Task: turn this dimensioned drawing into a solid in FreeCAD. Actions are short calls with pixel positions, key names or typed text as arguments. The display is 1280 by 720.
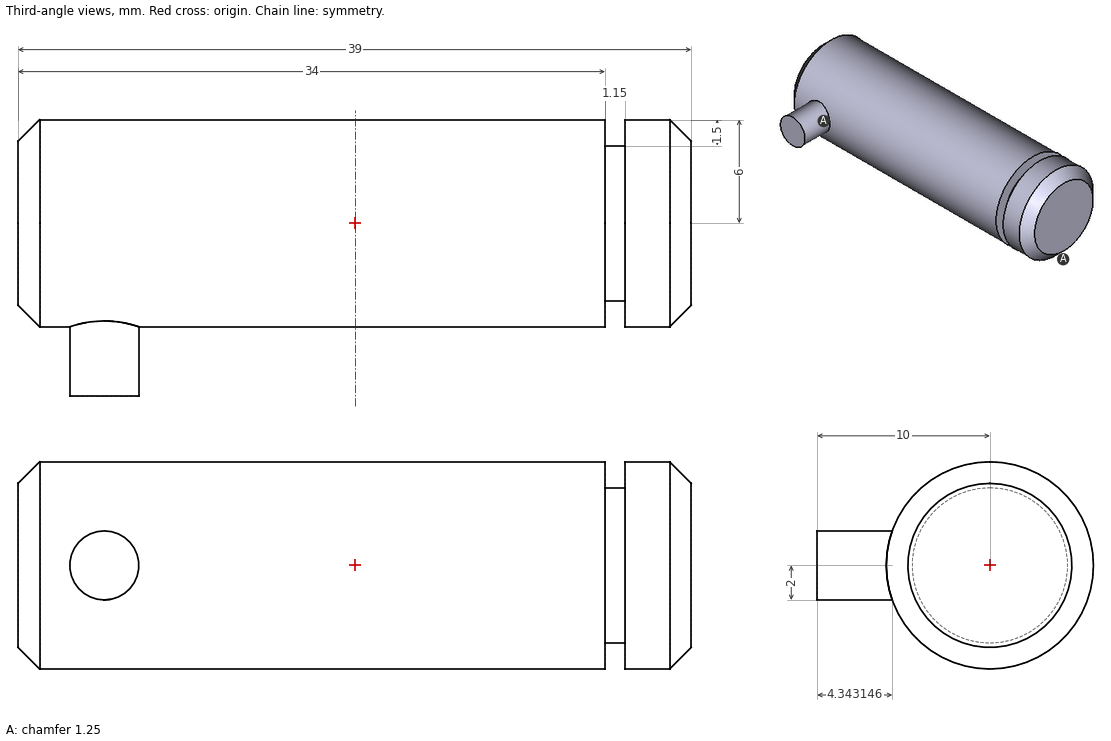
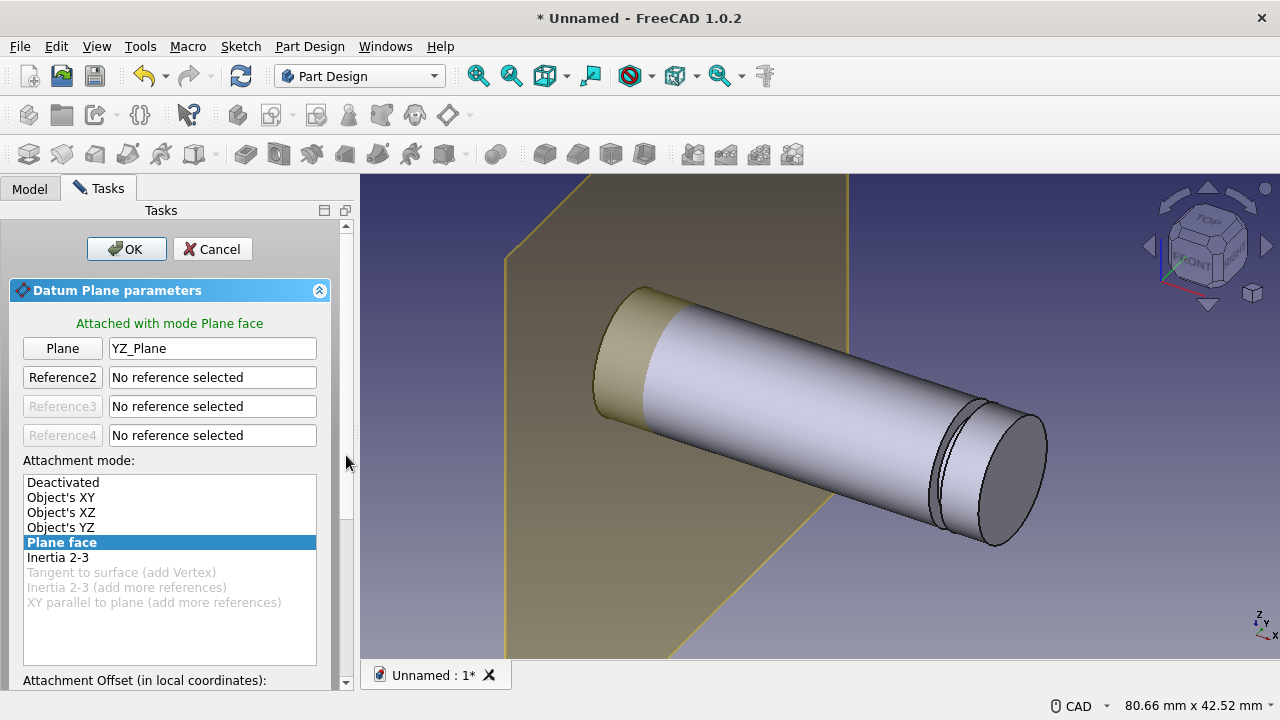
click(127, 249)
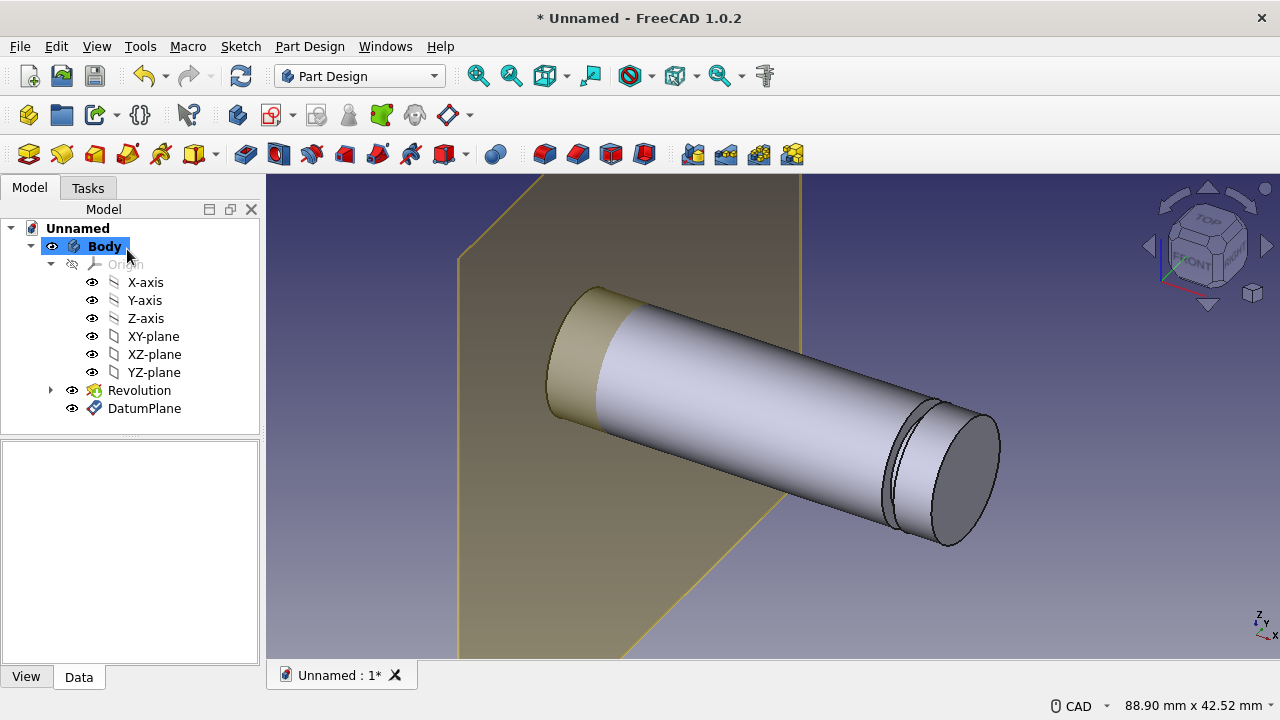
click(117, 408)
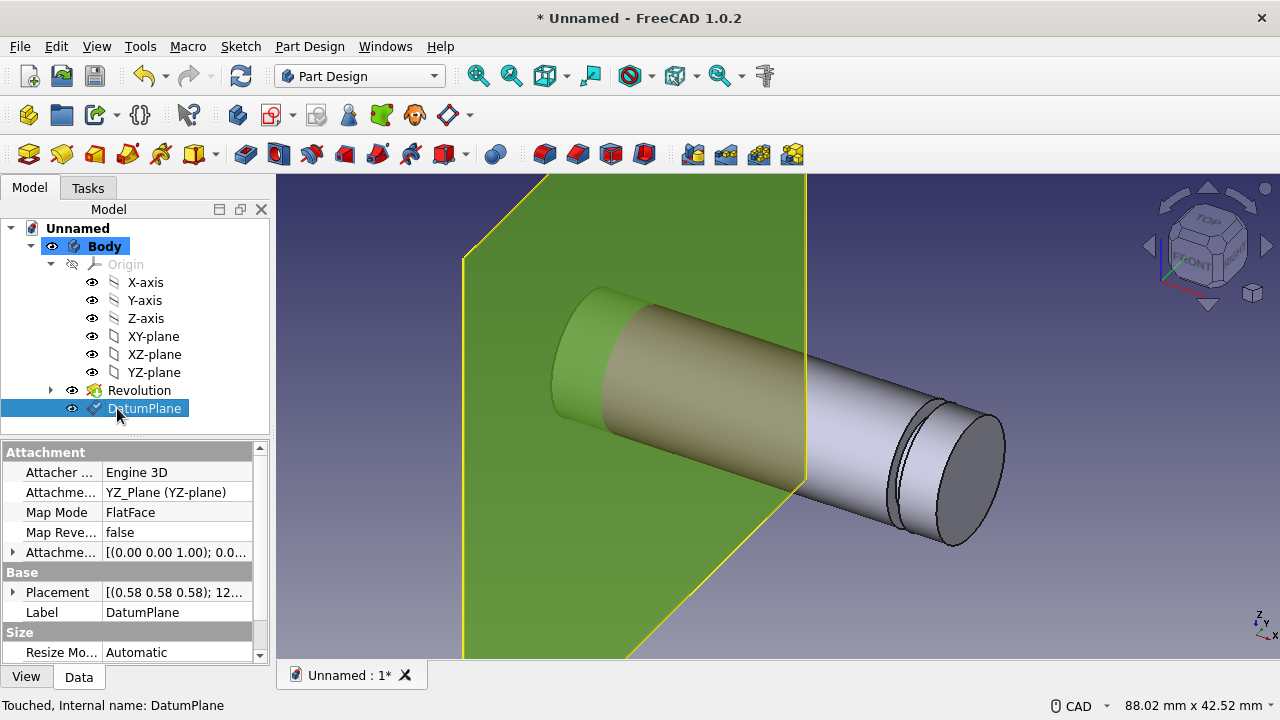
click(270, 116)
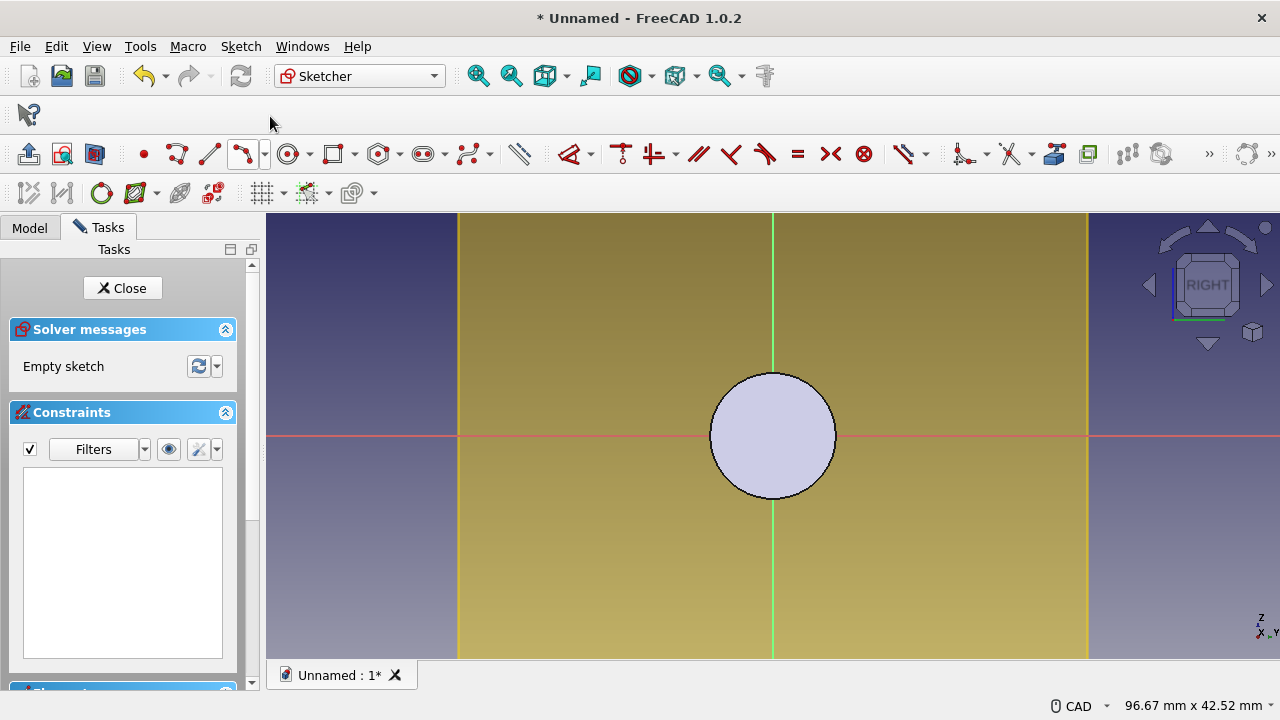
key(q)
key(s)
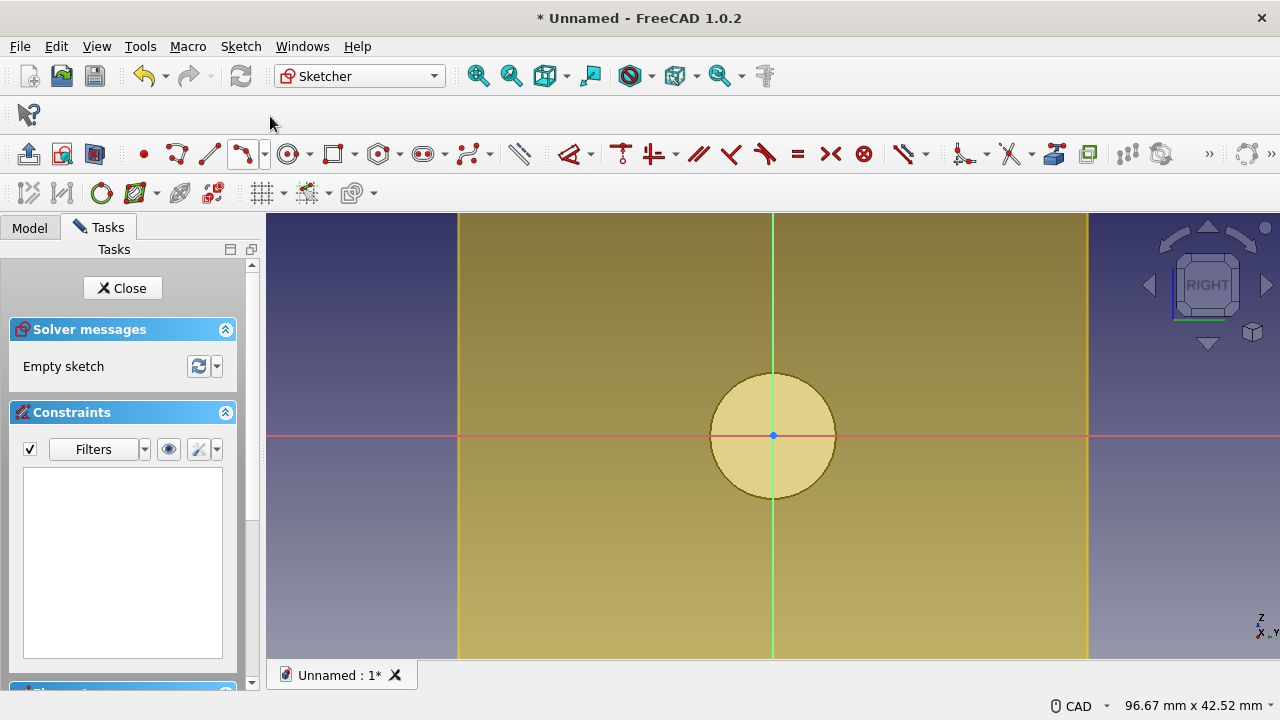
scroll(724, 449, up, 9)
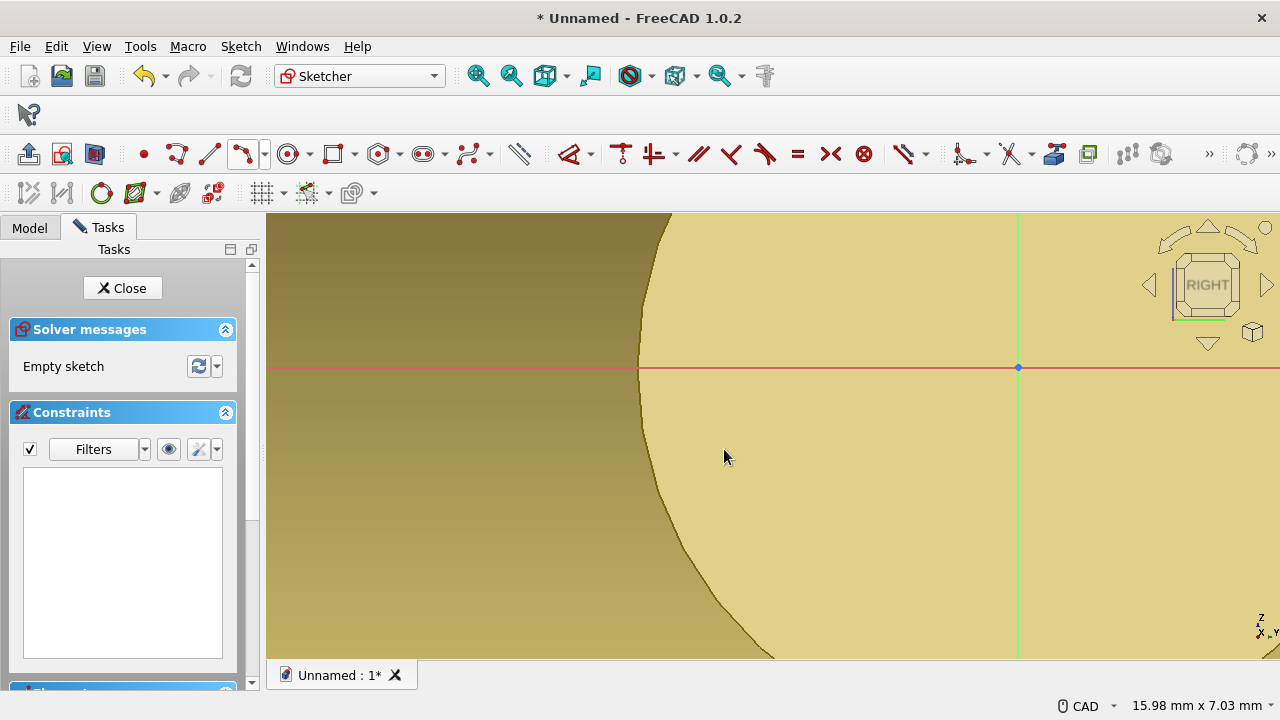
key(g)
key(r)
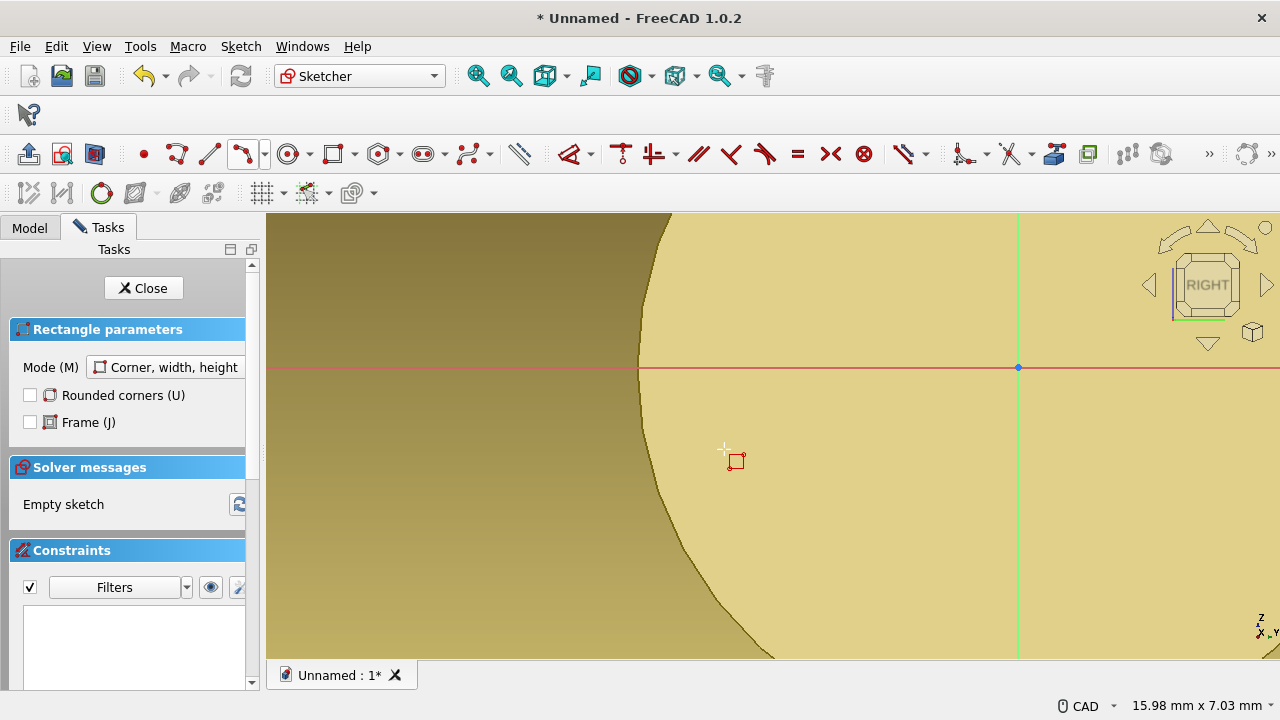
click(384, 368)
move(659, 495)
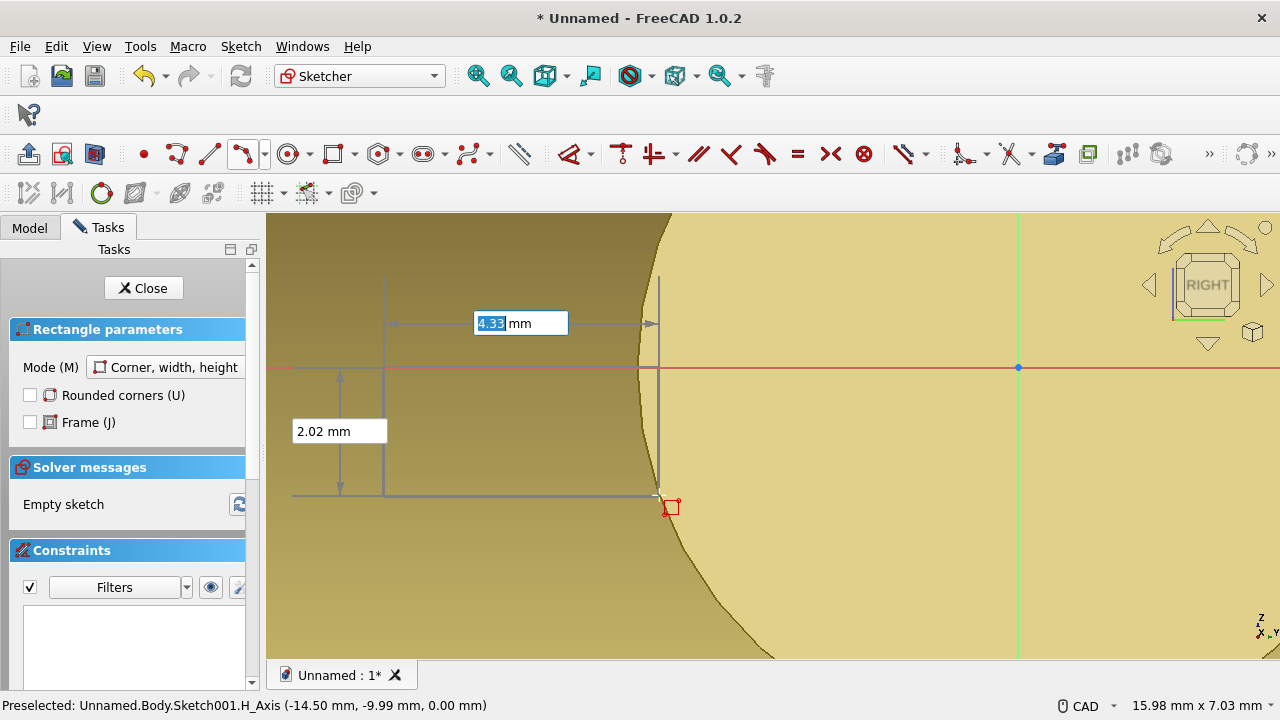
text(4.343146)
key(Tab)
text(2)
key(Return)
key(Escape)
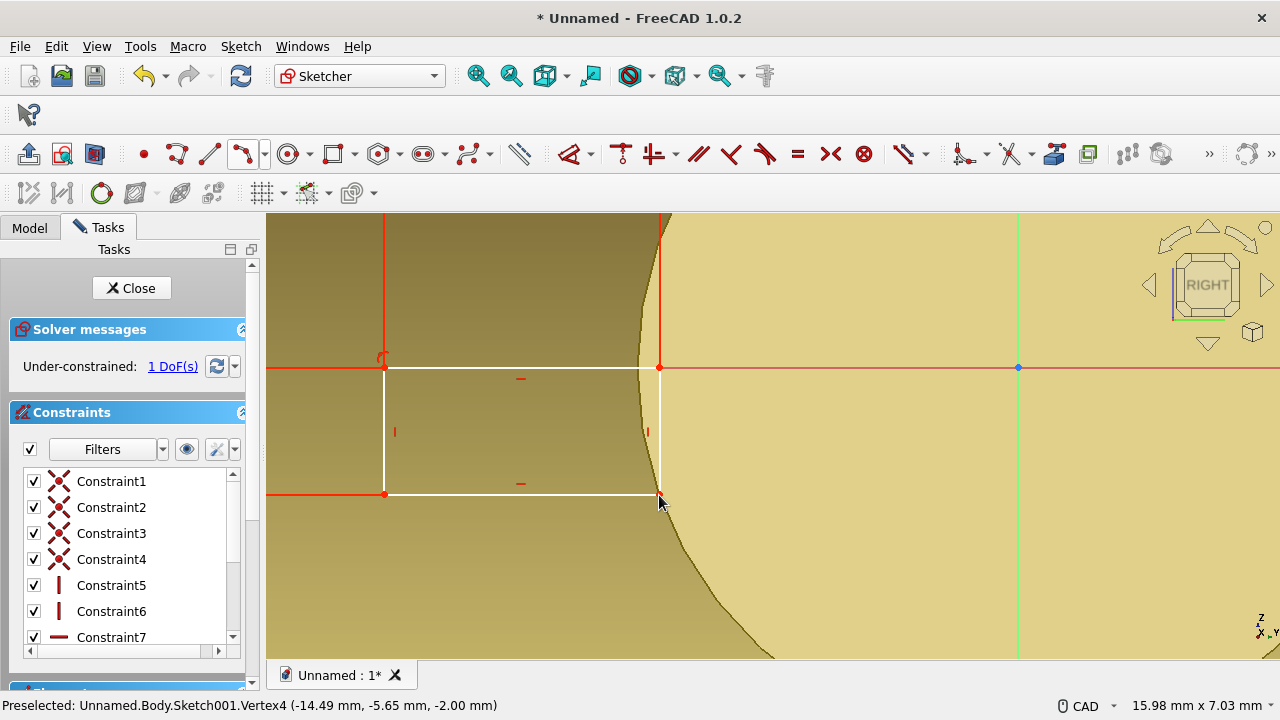
click(384, 368)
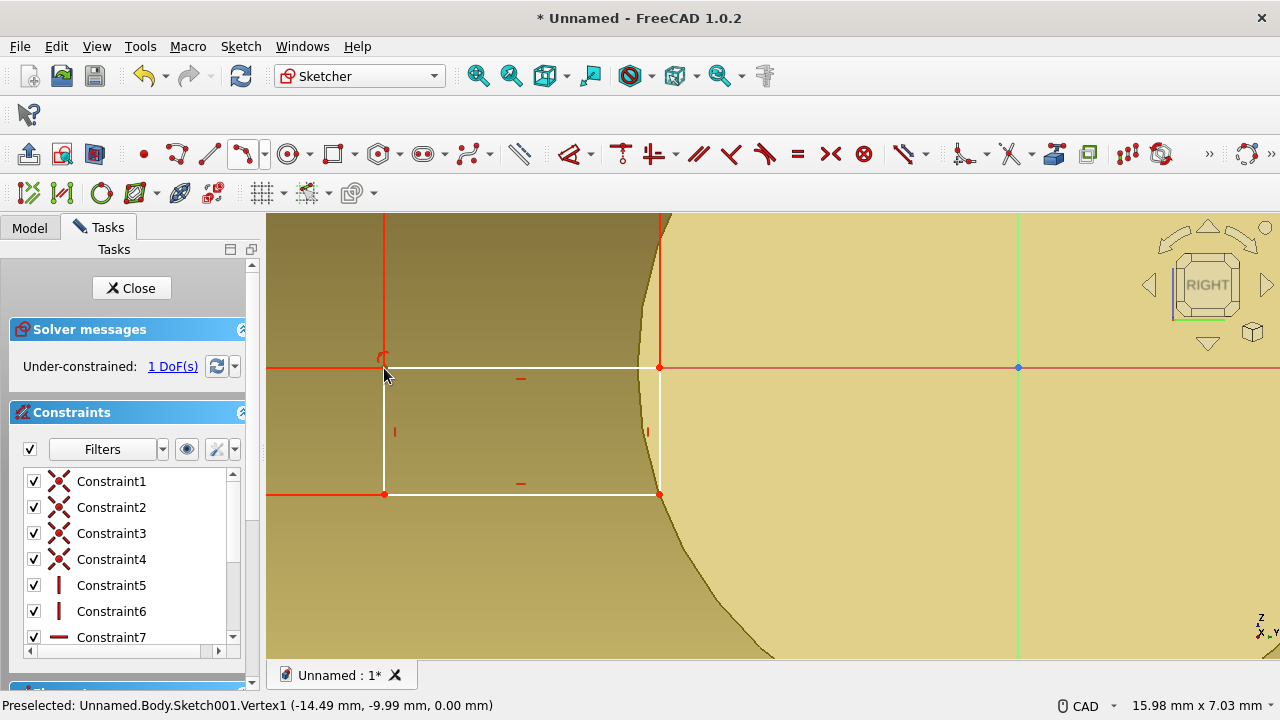
click(590, 154)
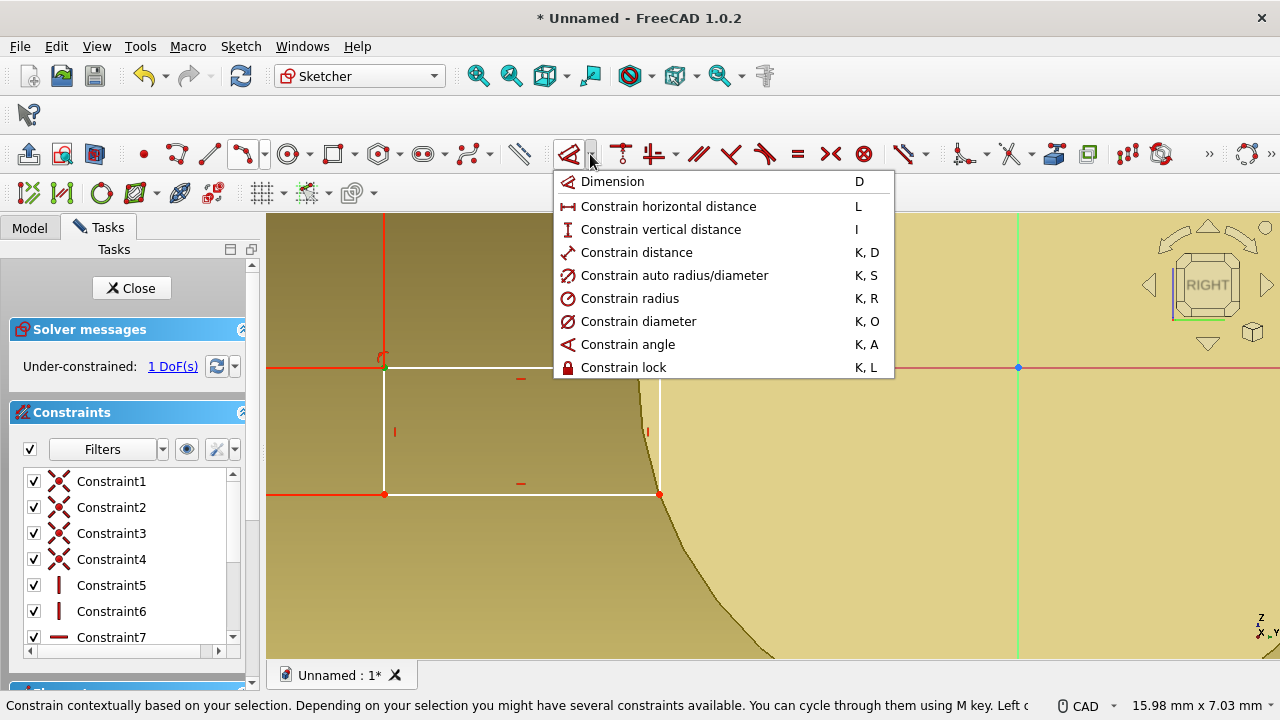
click(724, 206)